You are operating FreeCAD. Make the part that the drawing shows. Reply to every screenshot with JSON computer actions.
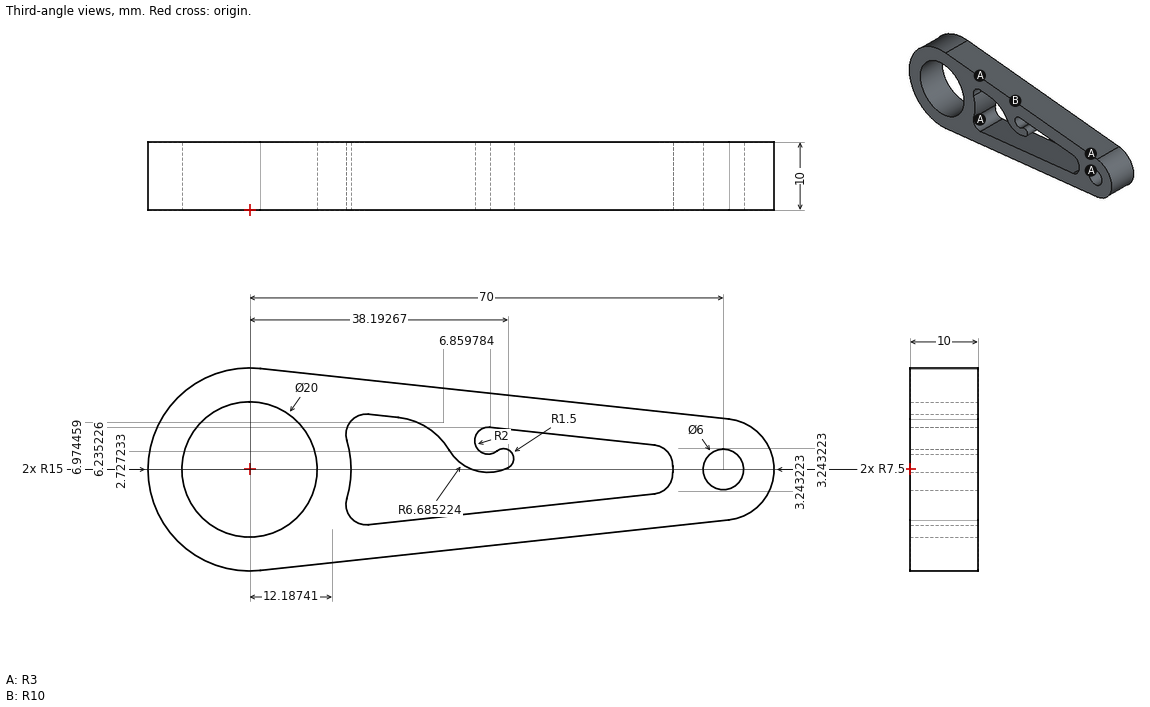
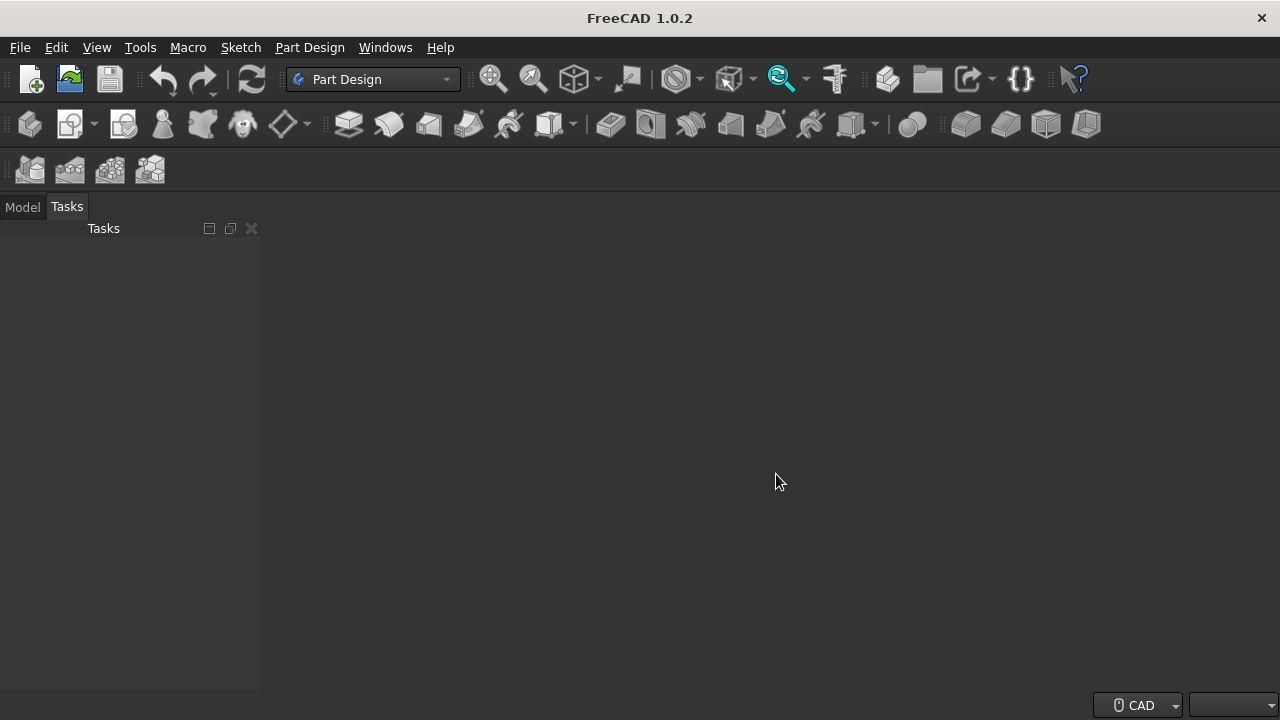
{"action": "left_click", "coordinate": [30, 80]}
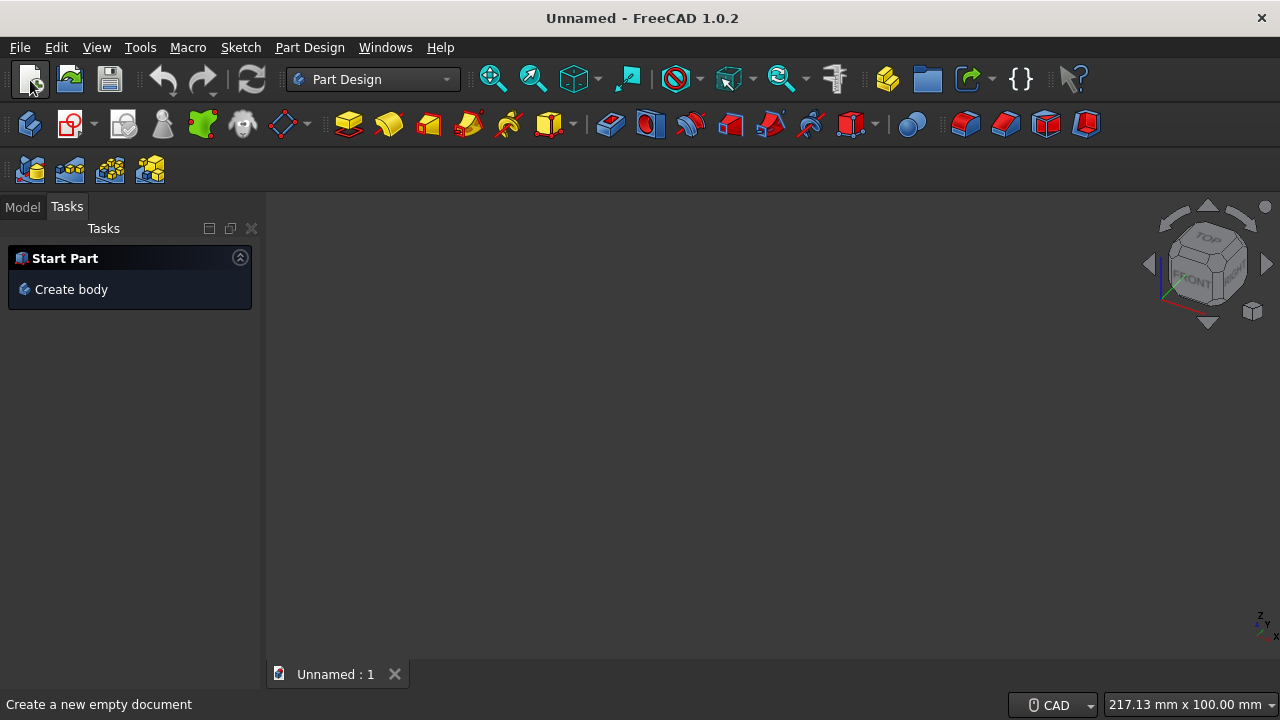
{"action": "left_click", "coordinate": [70, 124]}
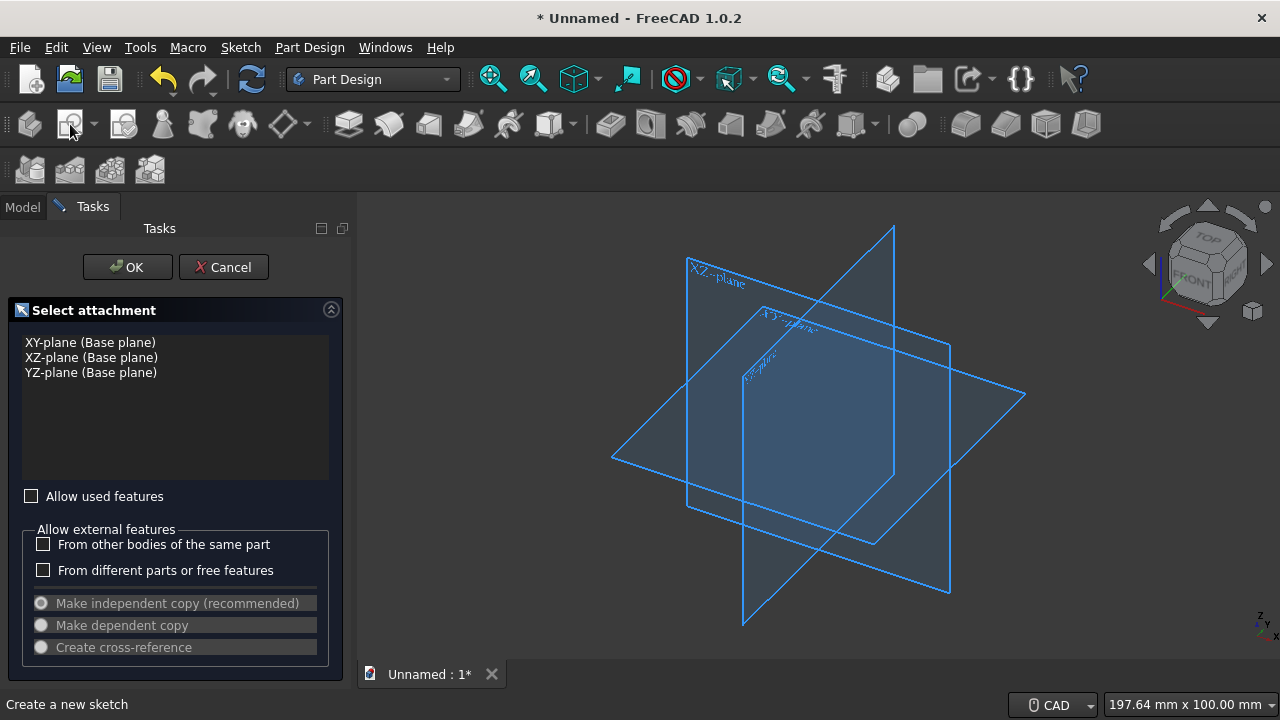
{"action": "left_click", "coordinate": [82, 358]}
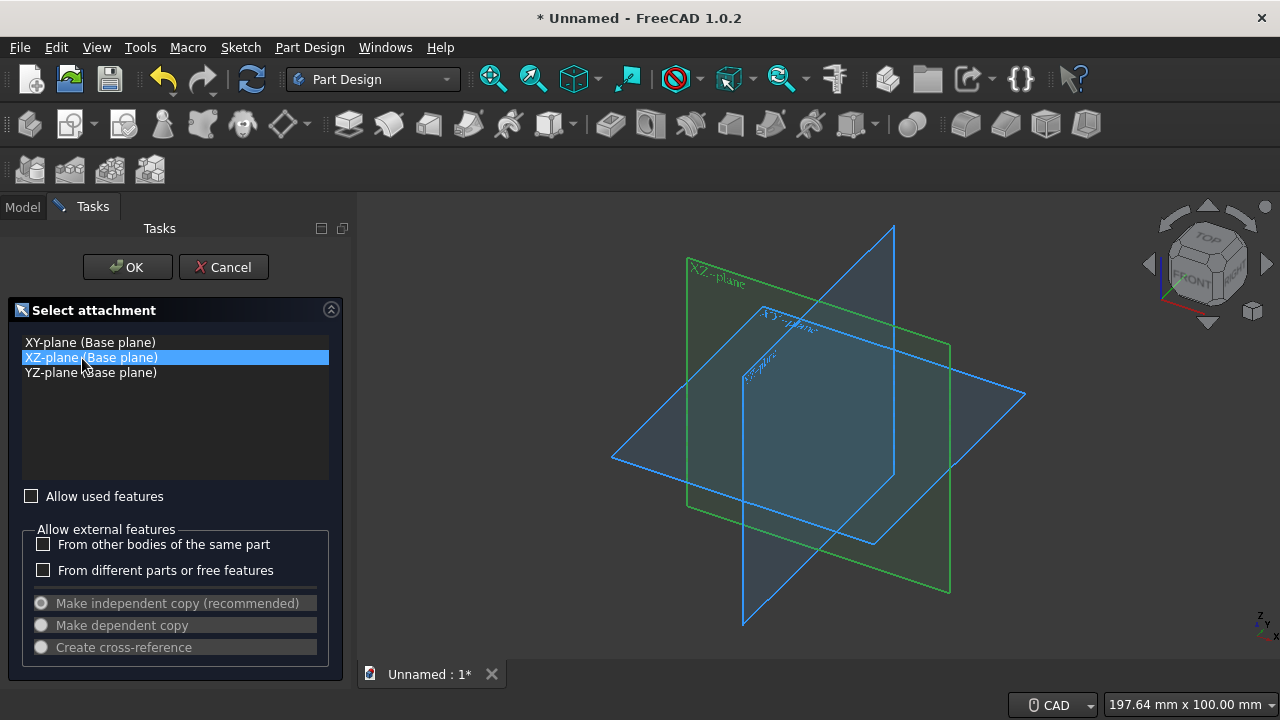
{"action": "left_click", "coordinate": [128, 267]}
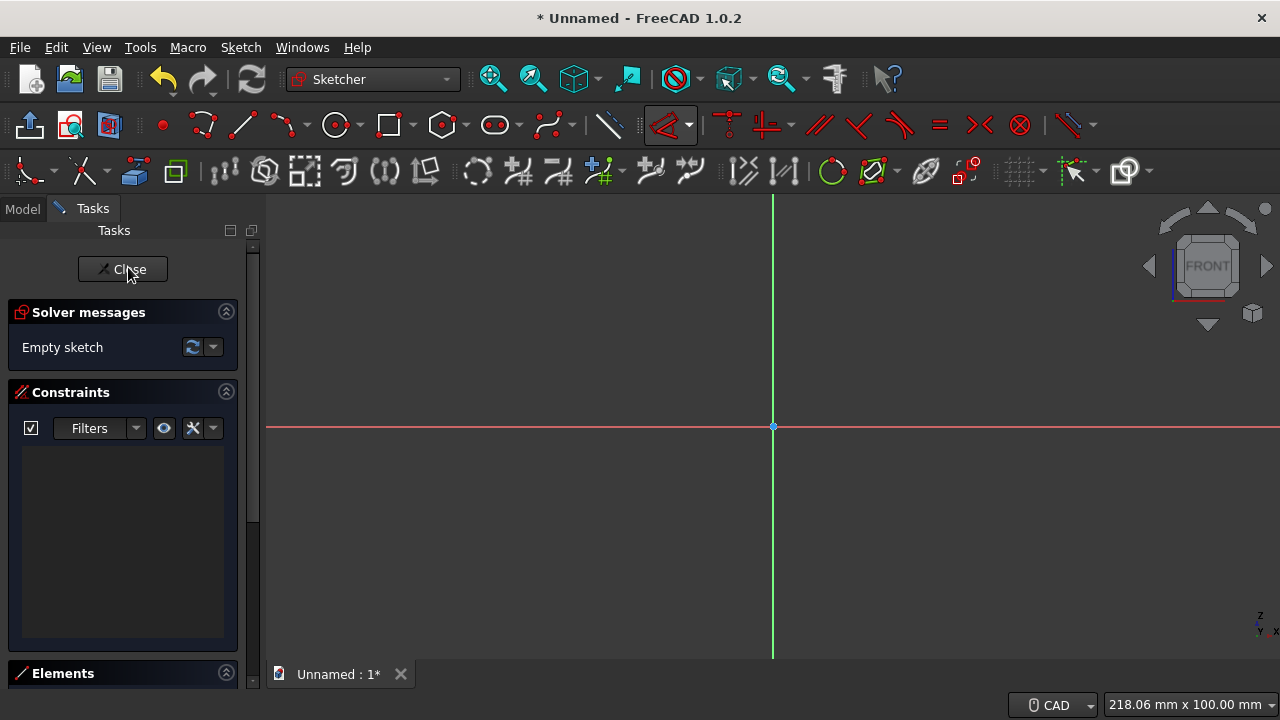
{"action": "scroll", "coordinate": [294, 427], "scroll_direction": "down", "scroll_amount": 1}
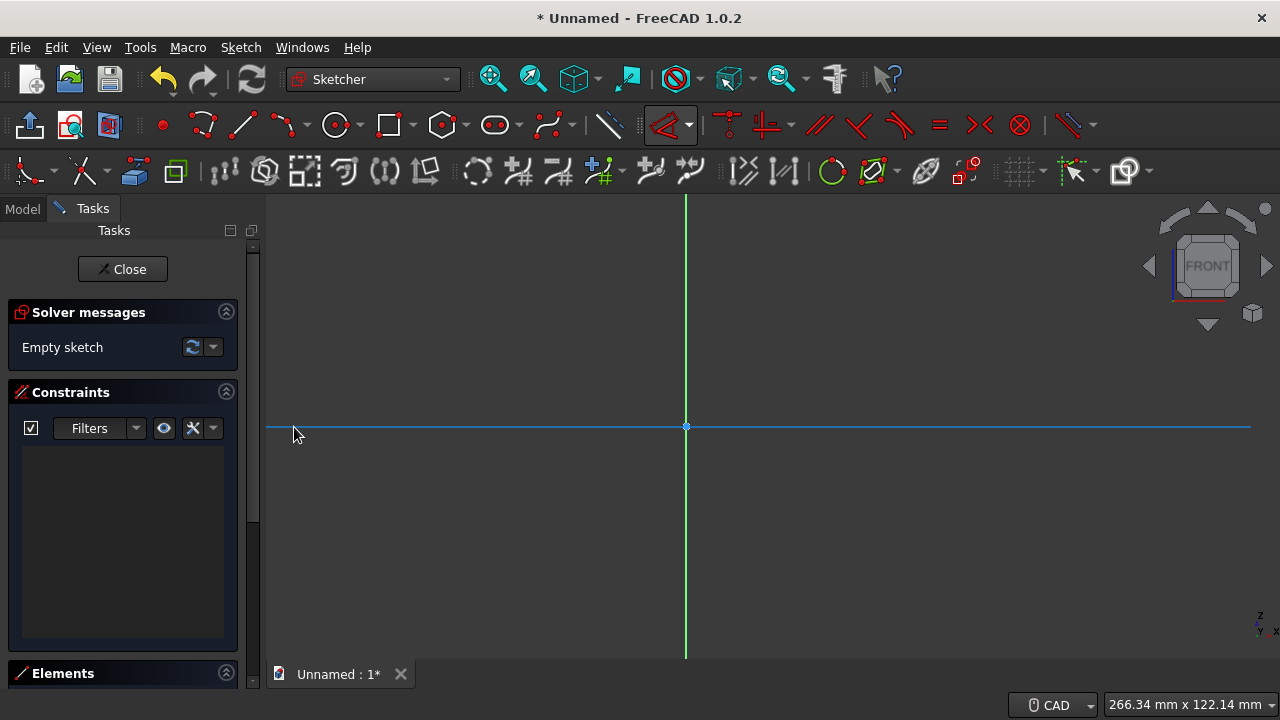
{"action": "scroll", "coordinate": [1010, 427], "scroll_direction": "up", "scroll_amount": 2}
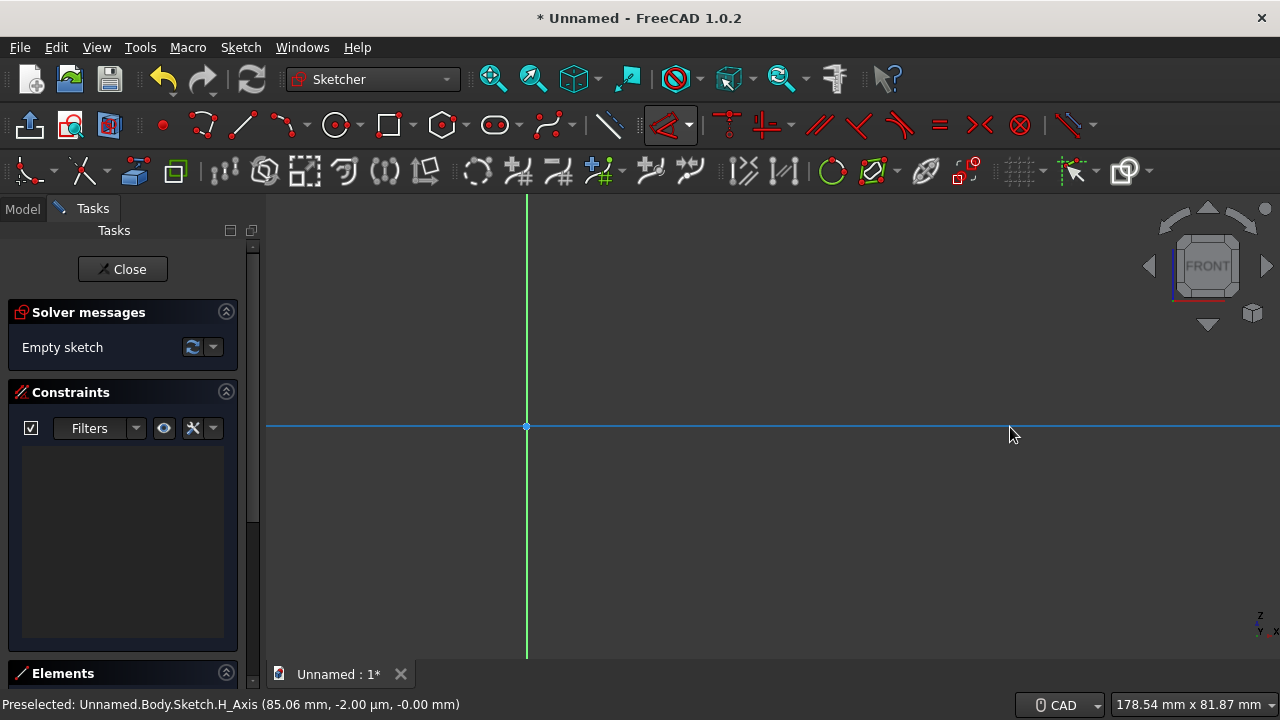
{"action": "left_click", "coordinate": [244, 126]}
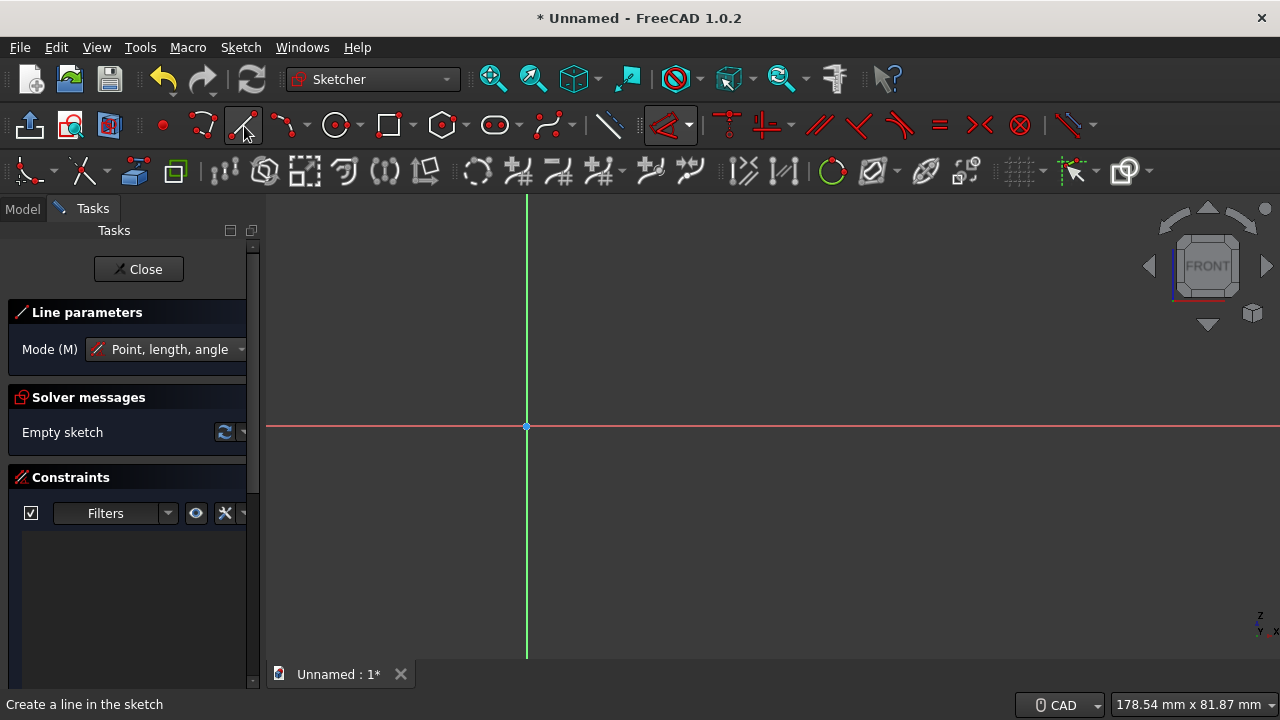
{"action": "left_click", "coordinate": [929, 469]}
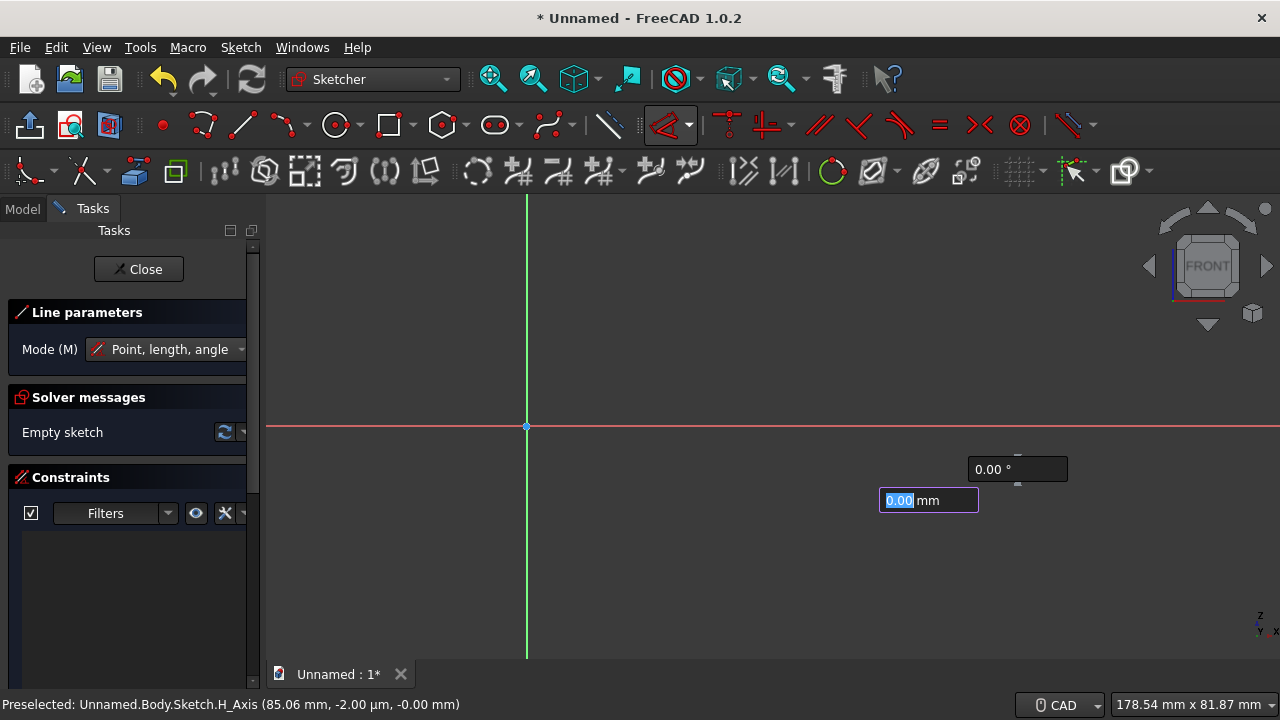
{"action": "scroll", "coordinate": [536, 511], "scroll_direction": "up", "scroll_amount": 3}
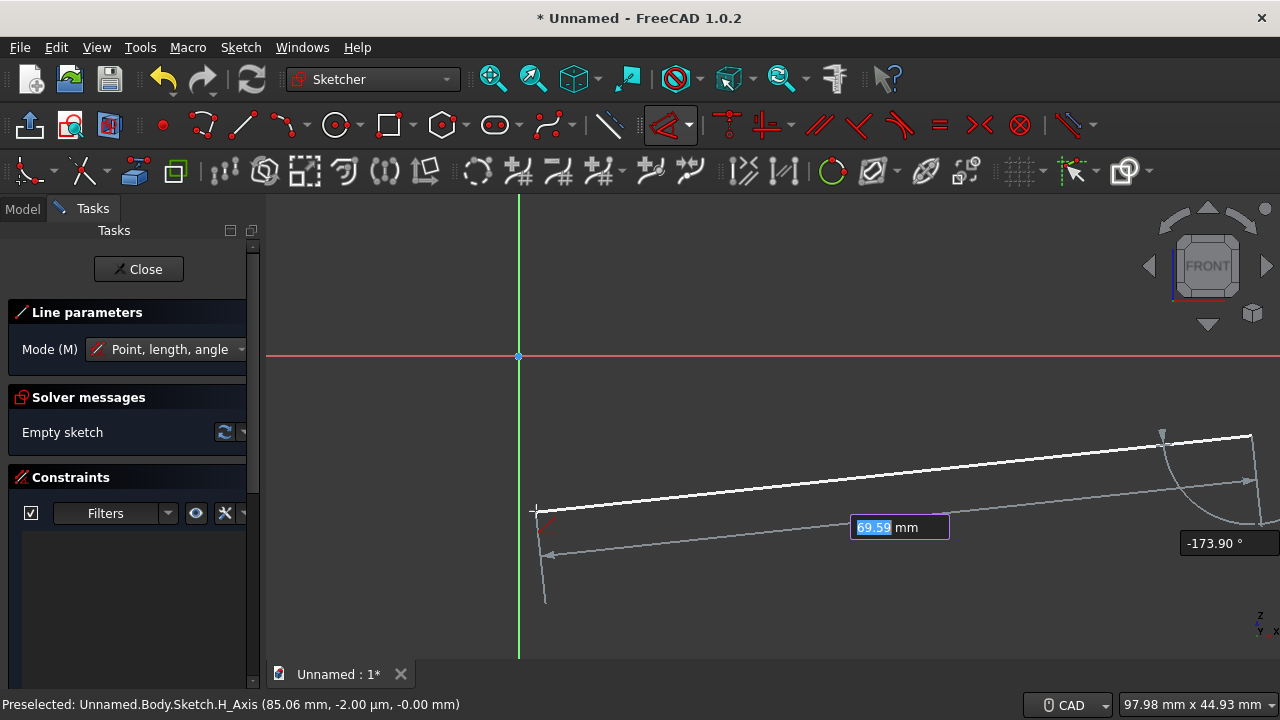
{"action": "left_click", "coordinate": [535, 510]}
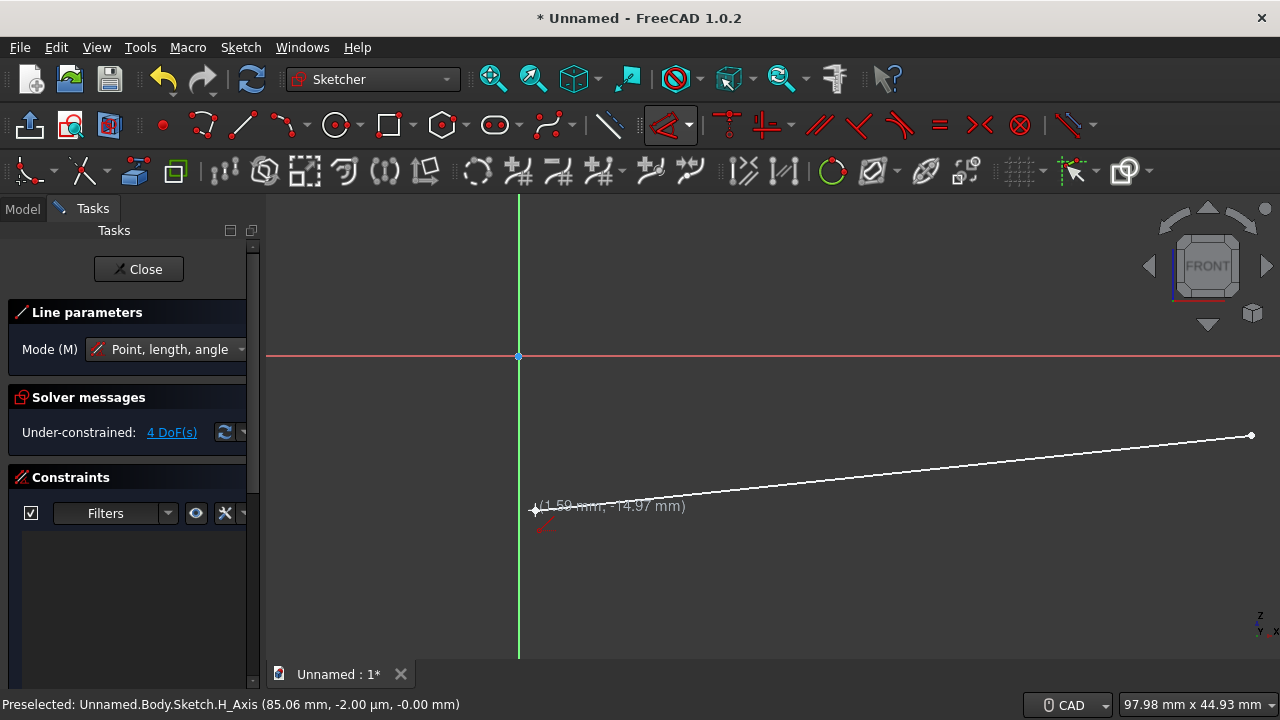
{"action": "scroll", "coordinate": [537, 512], "scroll_direction": "down", "scroll_amount": 3}